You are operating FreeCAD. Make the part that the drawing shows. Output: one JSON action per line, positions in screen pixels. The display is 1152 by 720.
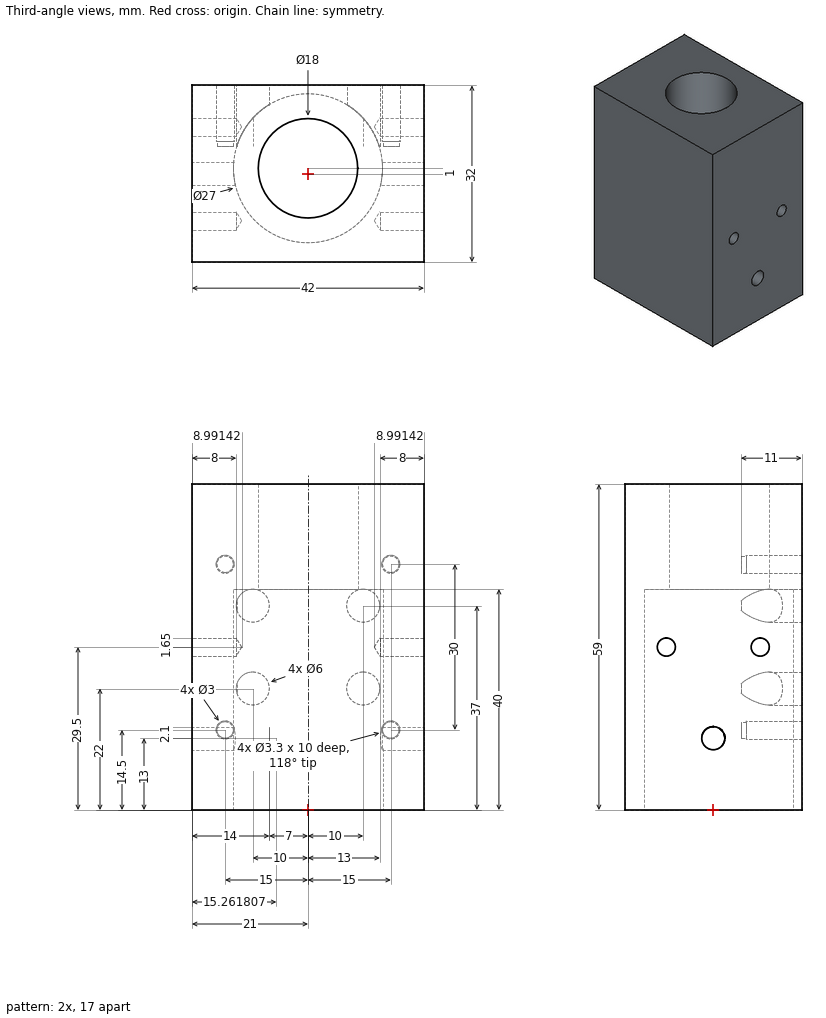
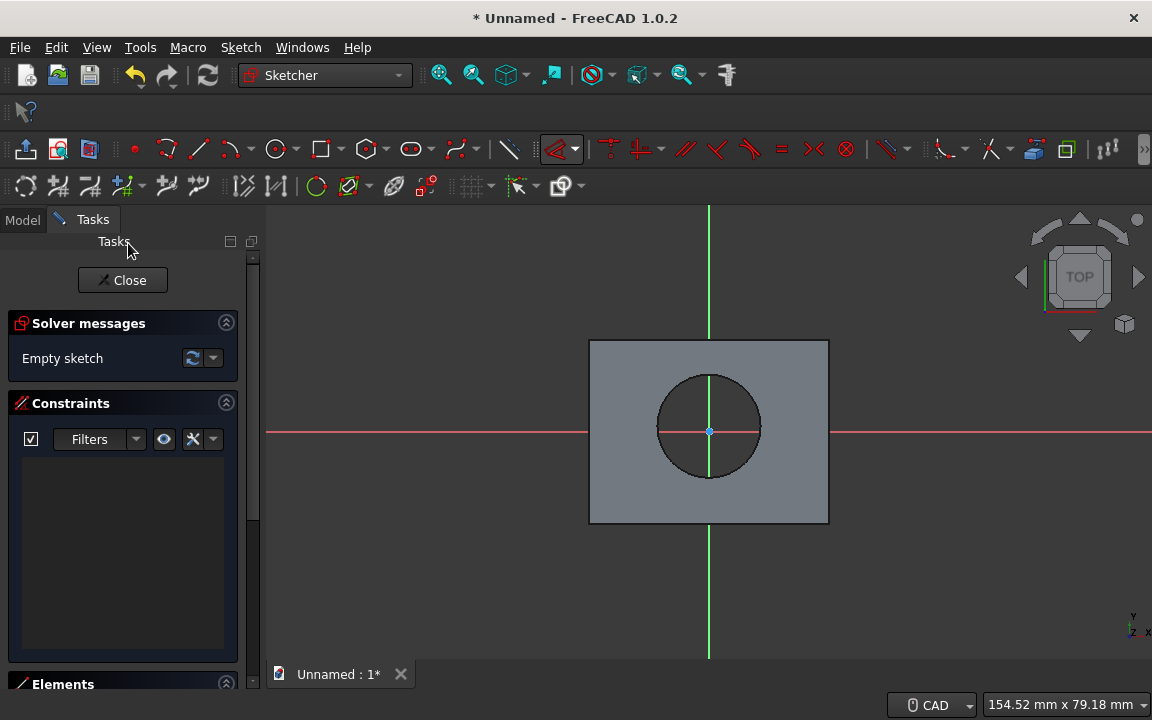
{"action": "left_click", "coordinate": [90, 150]}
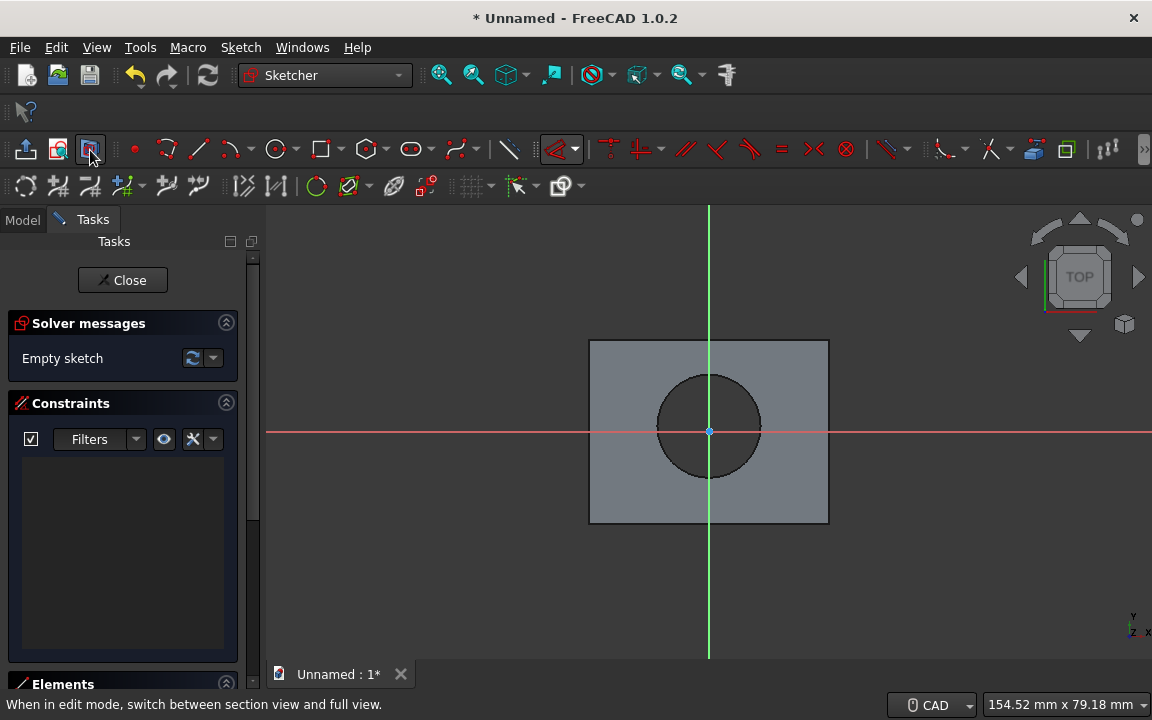
{"action": "scroll", "coordinate": [792, 419], "scroll_direction": "up", "scroll_amount": 3}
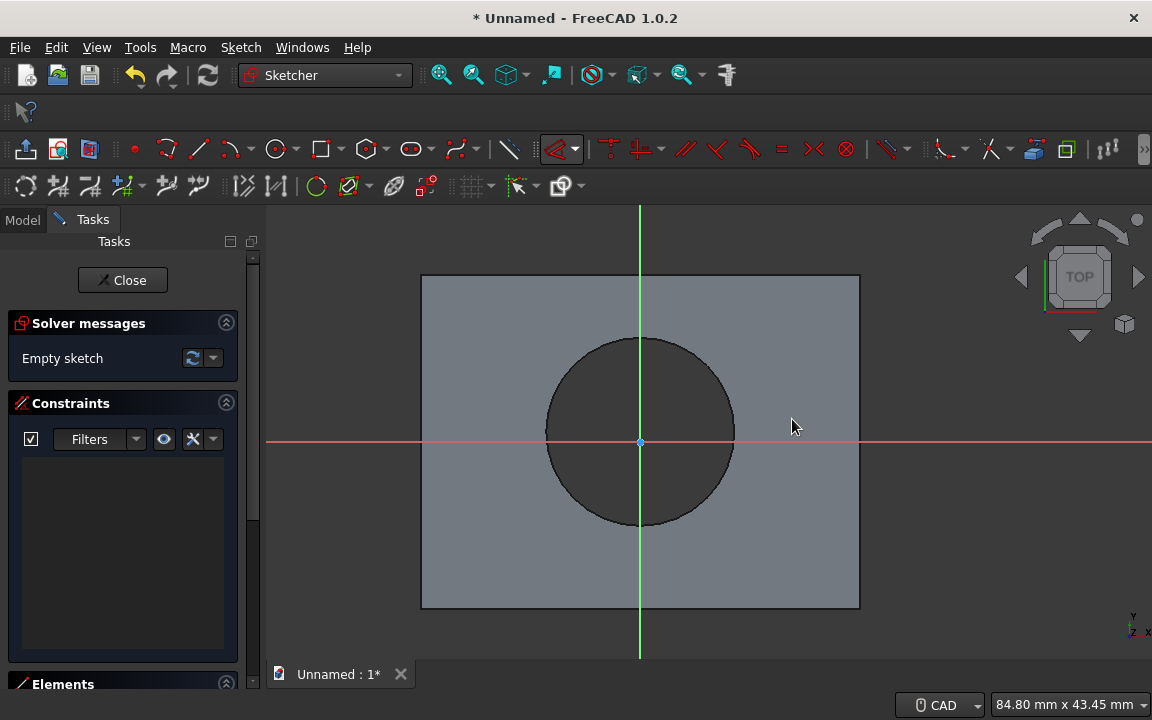
{"action": "left_click", "coordinate": [276, 150]}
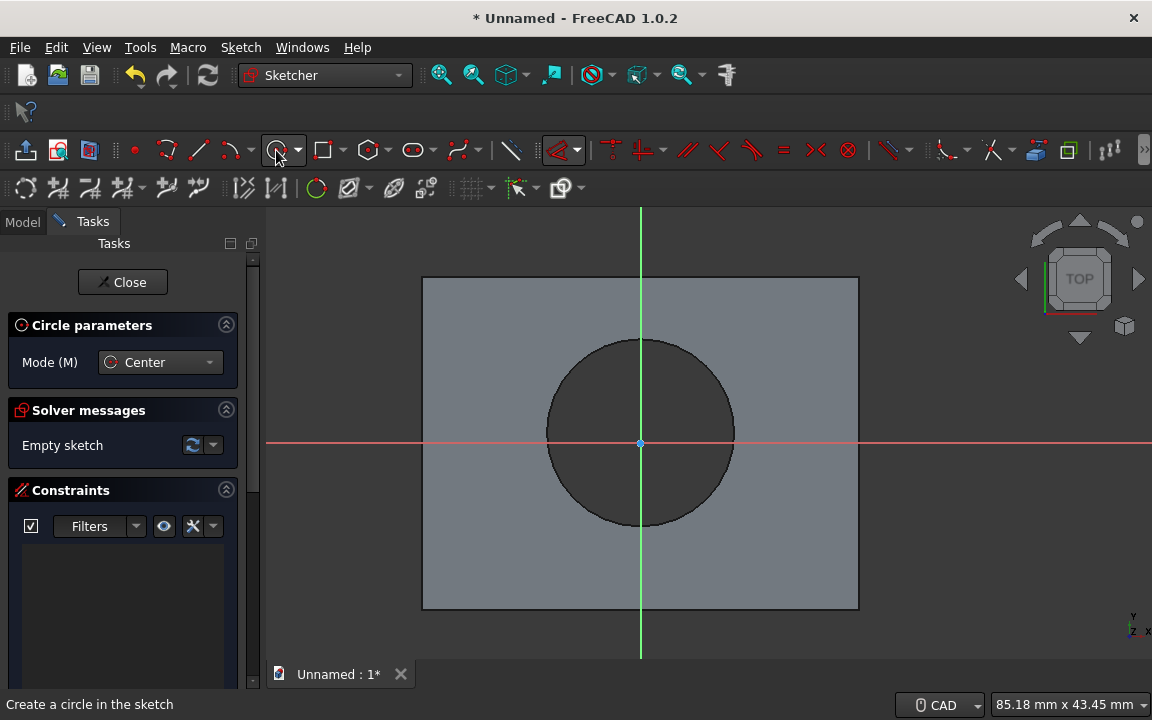
{"action": "scroll", "coordinate": [641, 433], "scroll_direction": "up", "scroll_amount": 3}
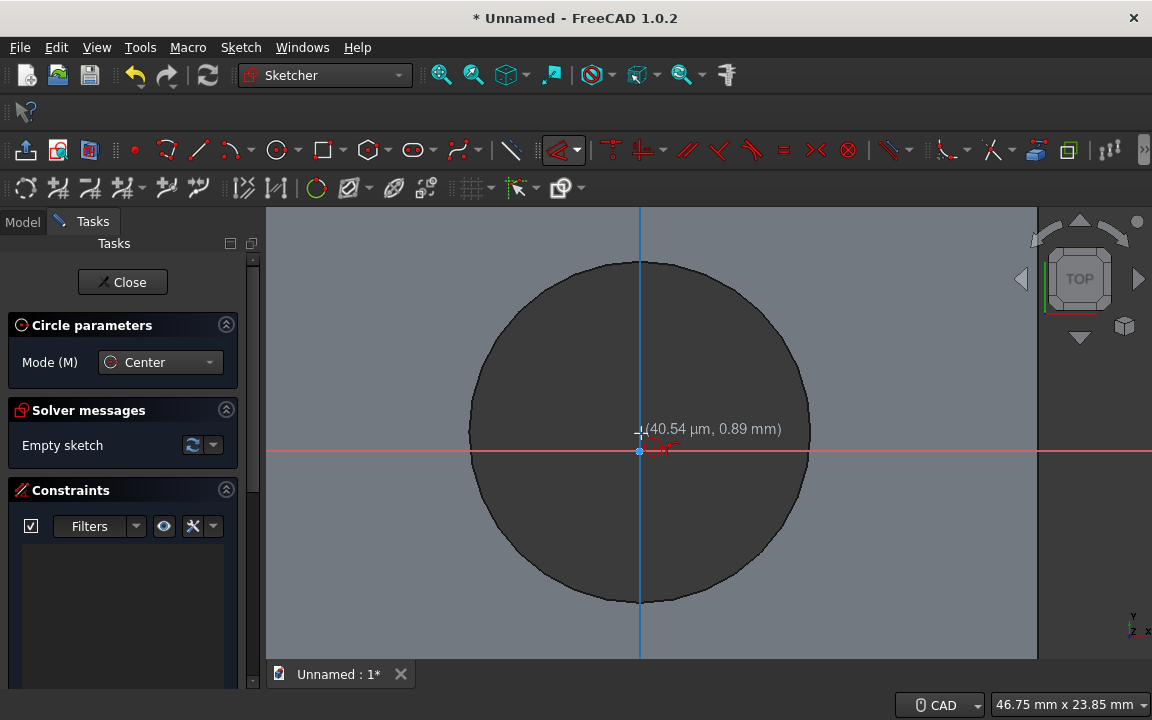
{"action": "left_click", "coordinate": [640, 432]}
{"action": "left_click", "coordinate": [821, 251]}
{"action": "key", "text": "Escape"}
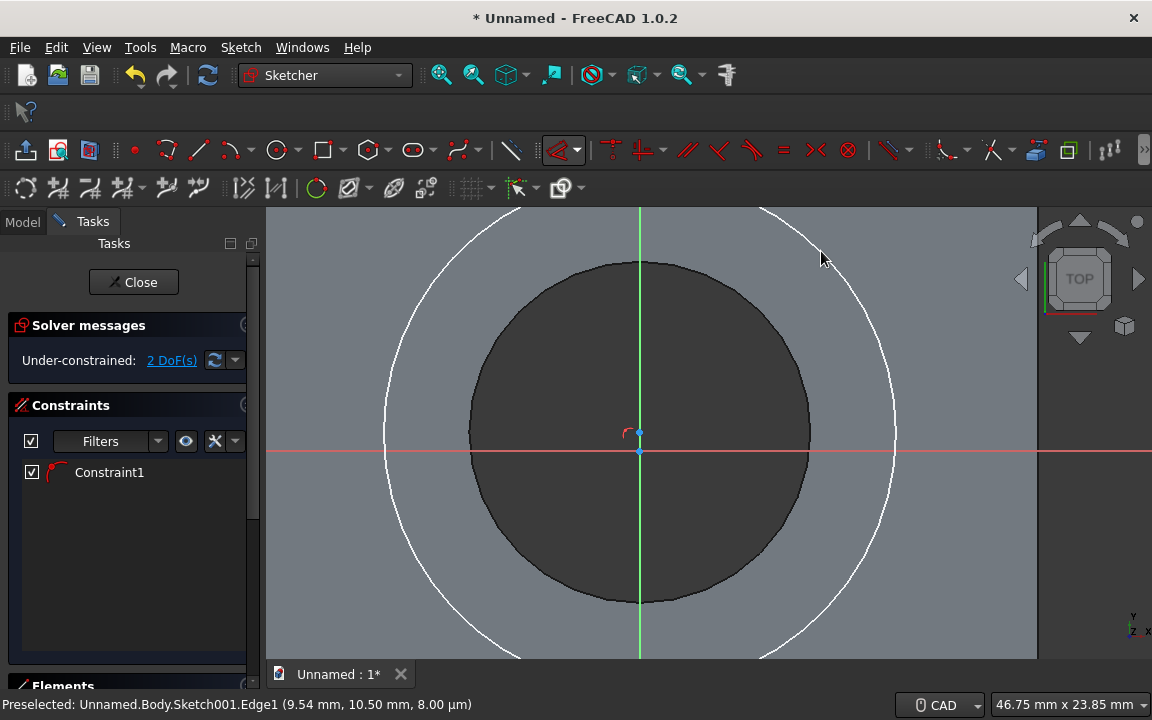
{"action": "left_click", "coordinate": [820, 251]}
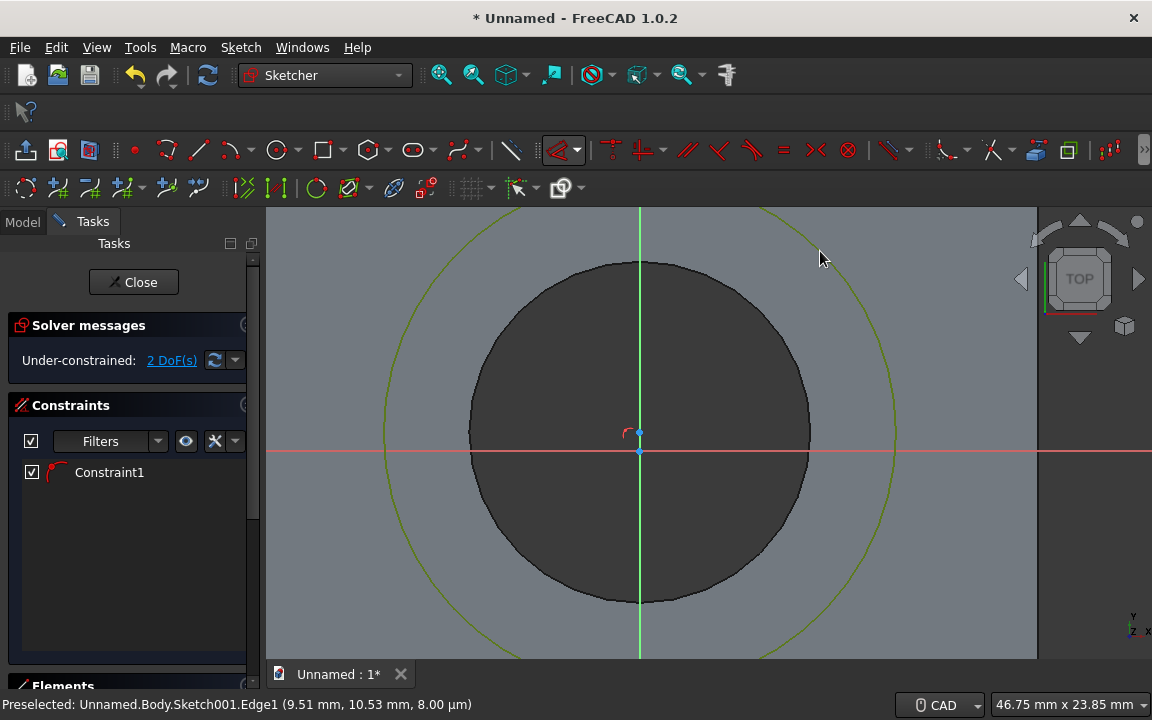
{"action": "key", "text": "k o"}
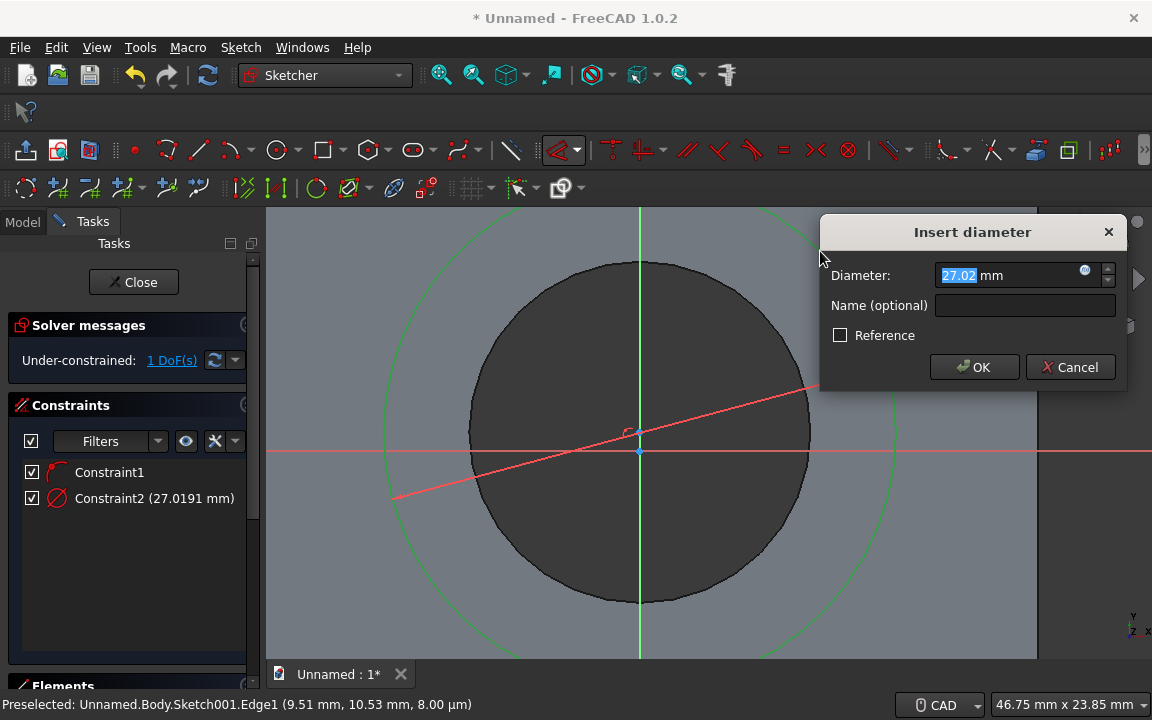
{"action": "type", "text": "27"}
{"action": "key", "text": "Return"}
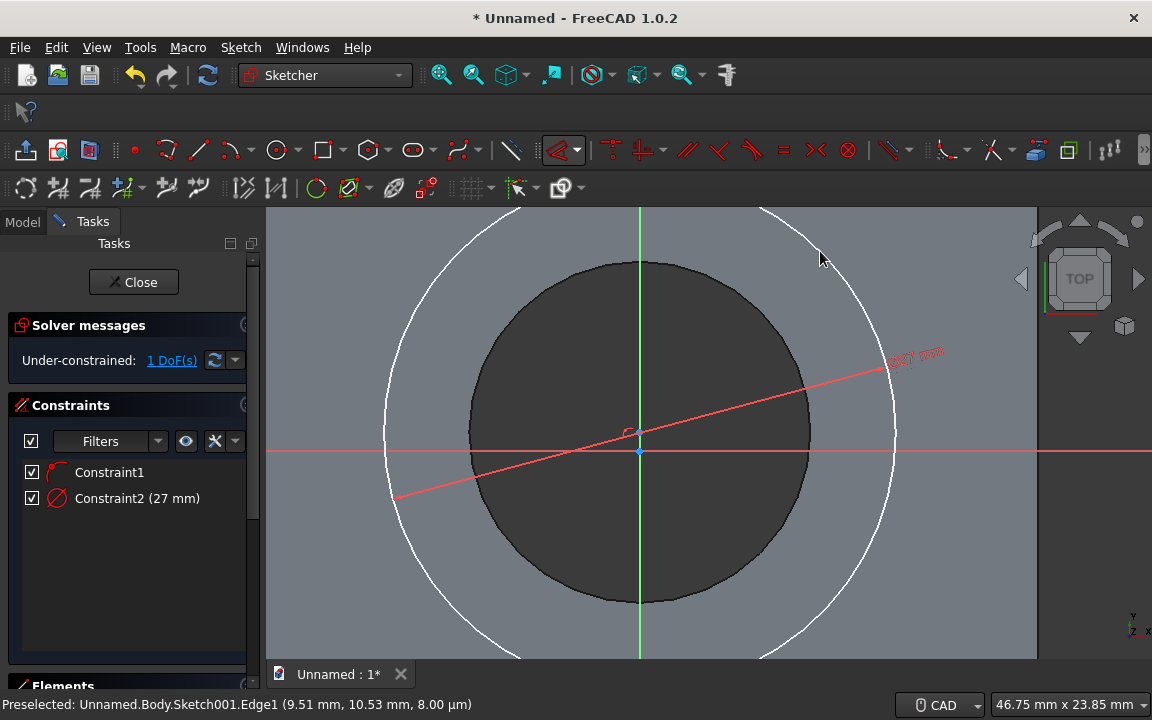
{"action": "scroll", "coordinate": [640, 433], "scroll_direction": "up", "scroll_amount": 4}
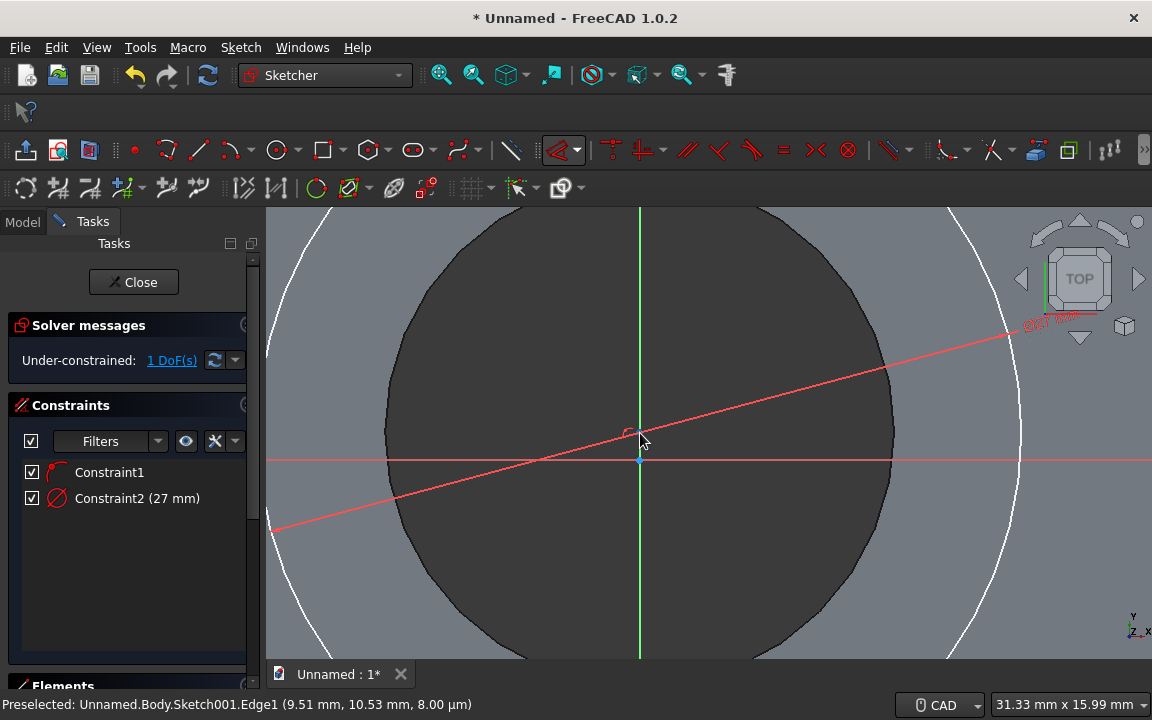
{"action": "left_click", "coordinate": [639, 432]}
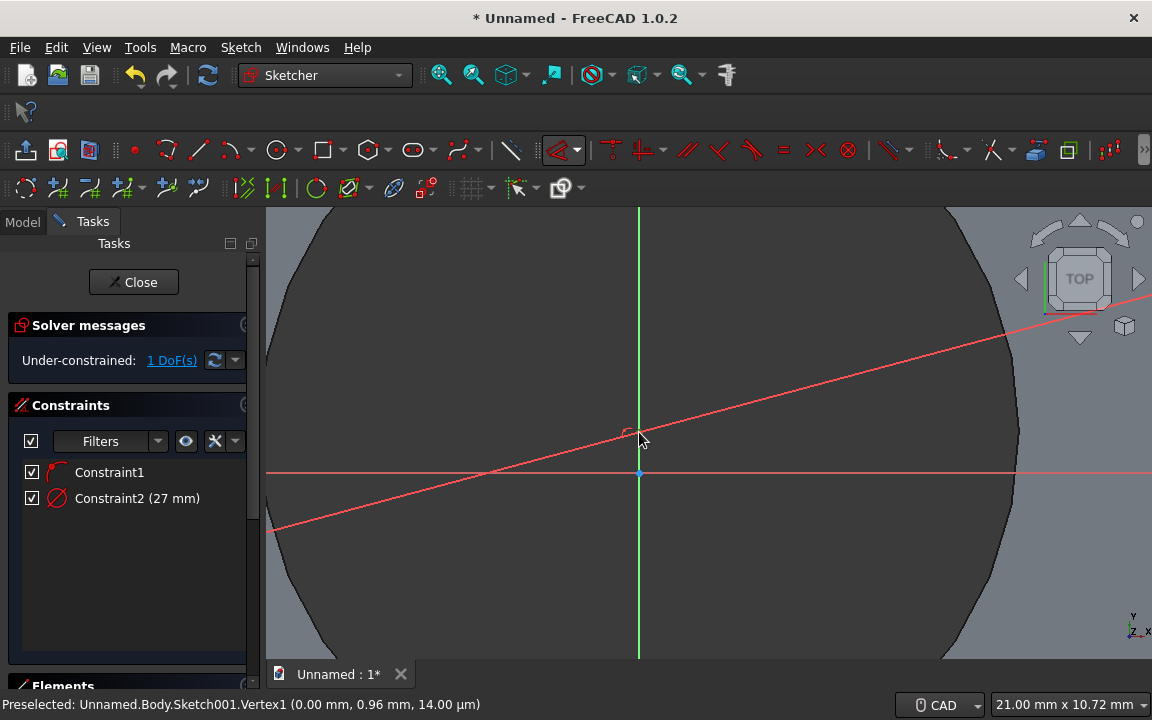
{"action": "key", "text": "i"}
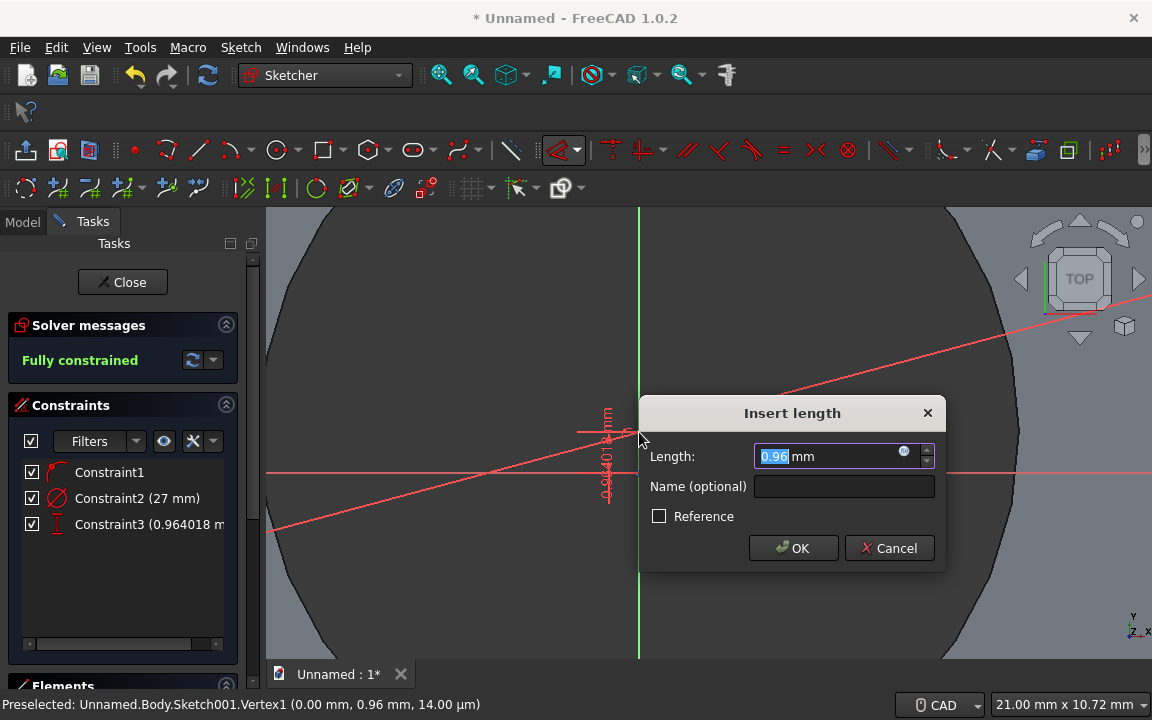
{"action": "type", "text": "1"}
{"action": "key", "text": "Return"}